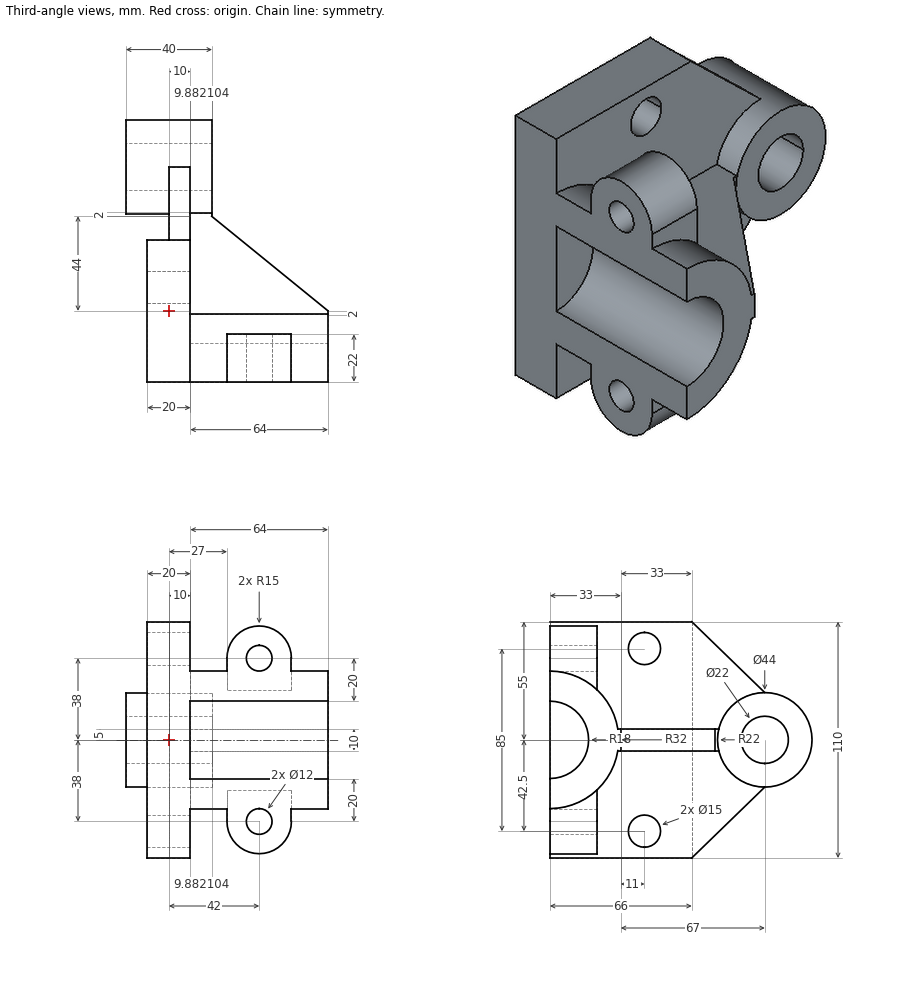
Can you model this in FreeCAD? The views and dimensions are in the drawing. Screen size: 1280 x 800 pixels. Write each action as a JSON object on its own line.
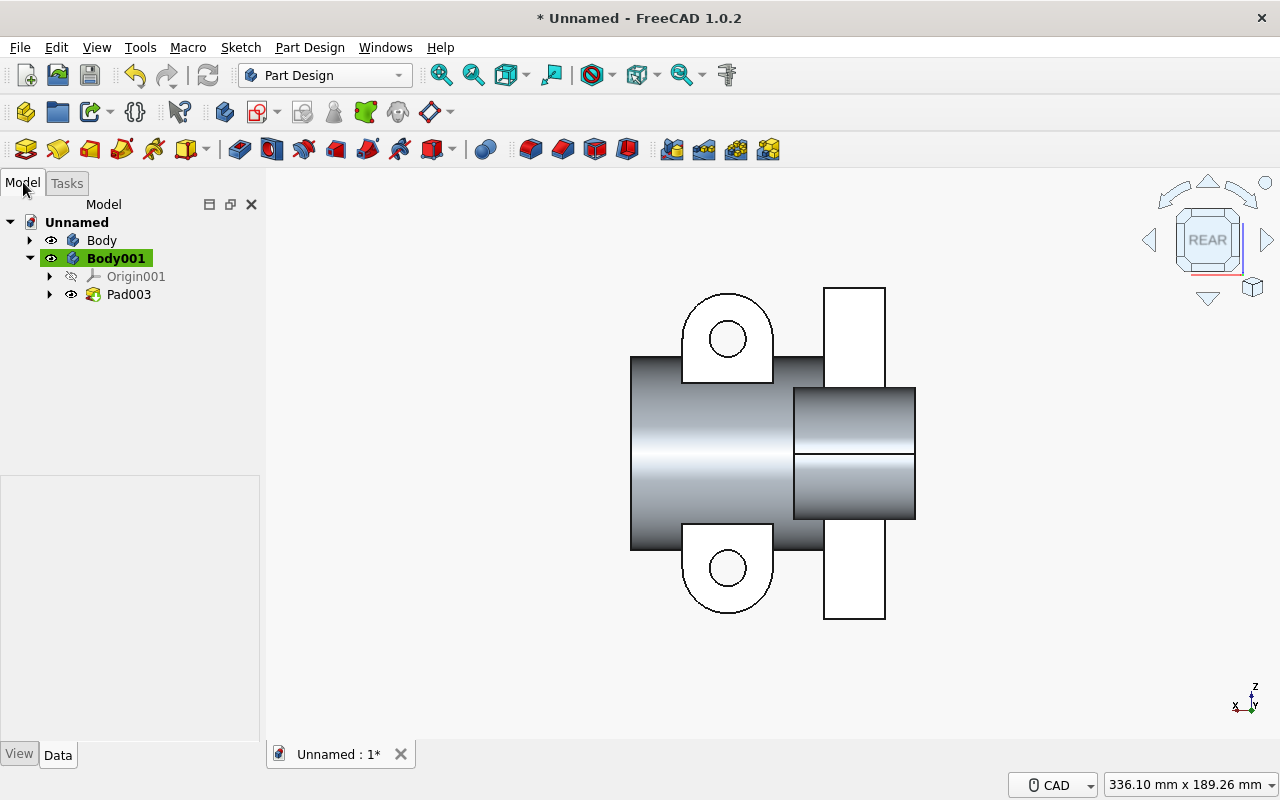
{"action": "double_click", "coordinate": [96, 240]}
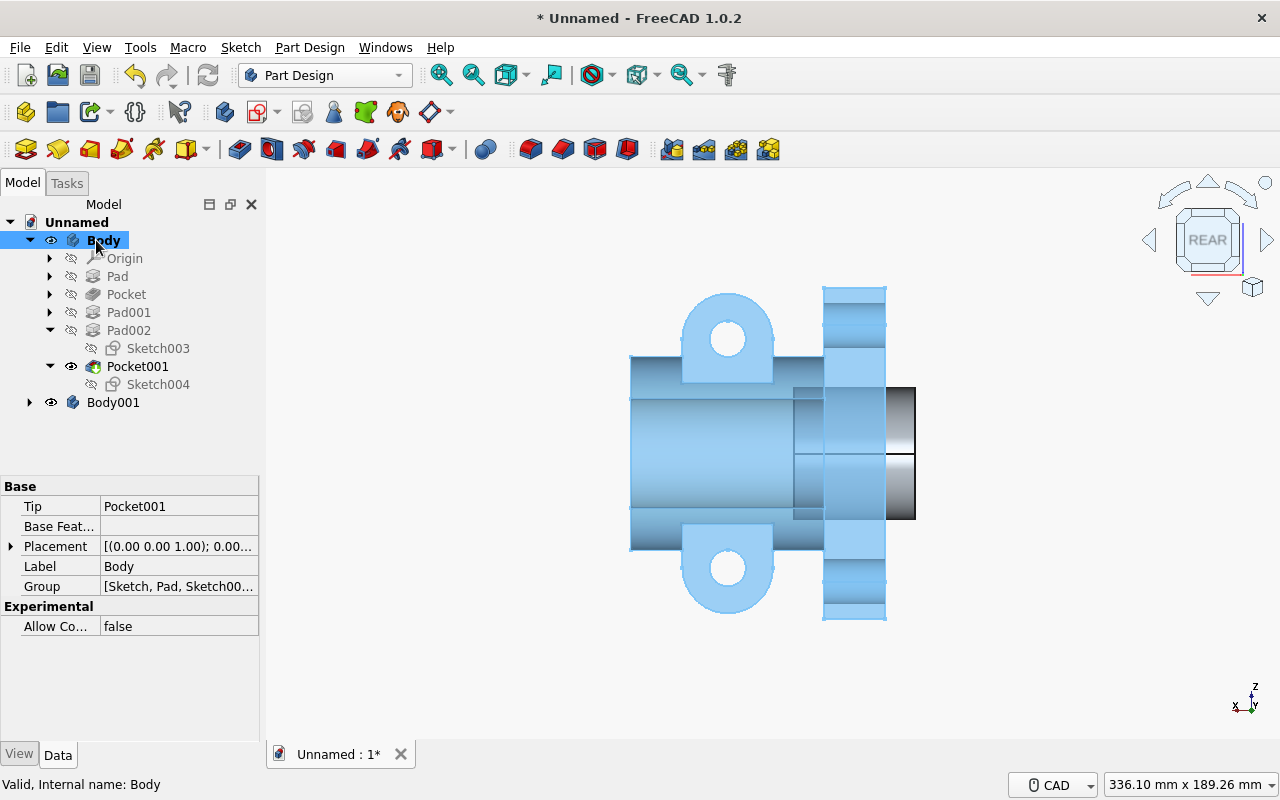
{"action": "left_click", "coordinate": [96, 240]}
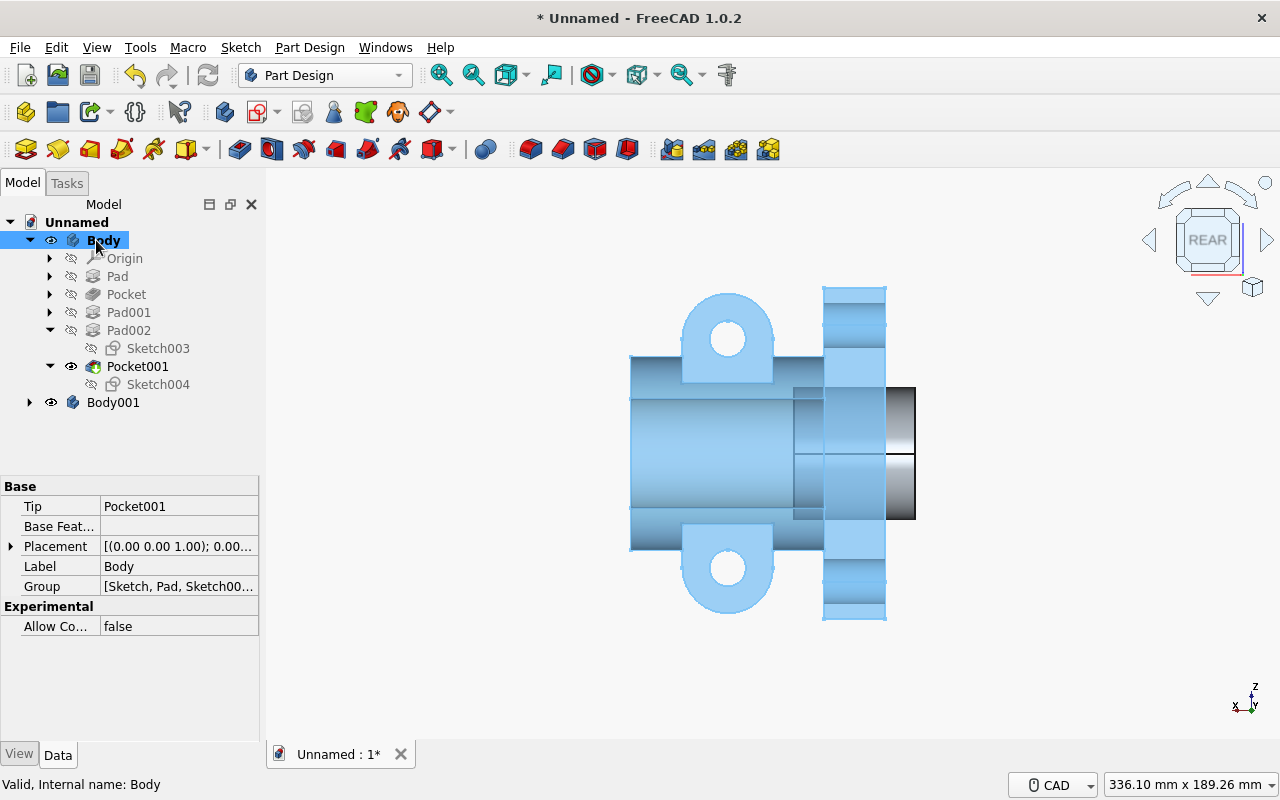
{"action": "left_click", "coordinate": [146, 626]}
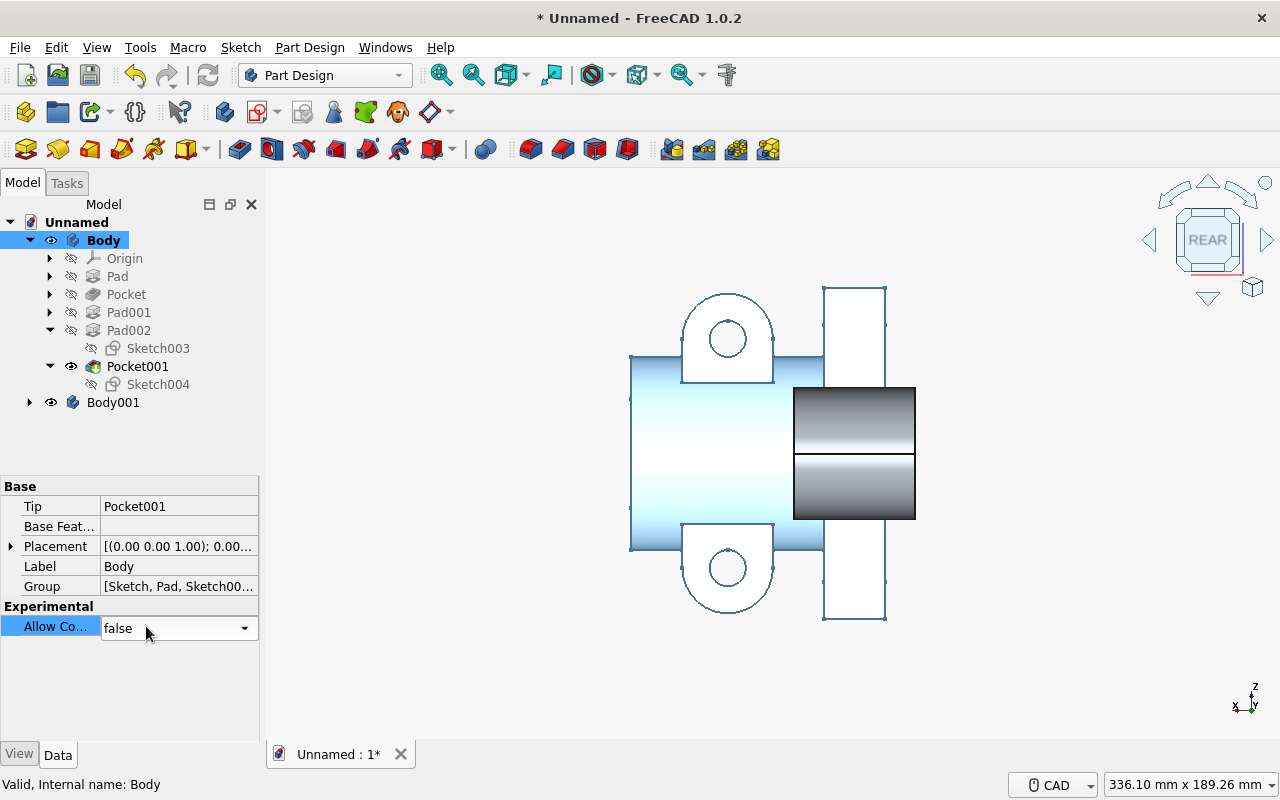
{"action": "left_click", "coordinate": [146, 626]}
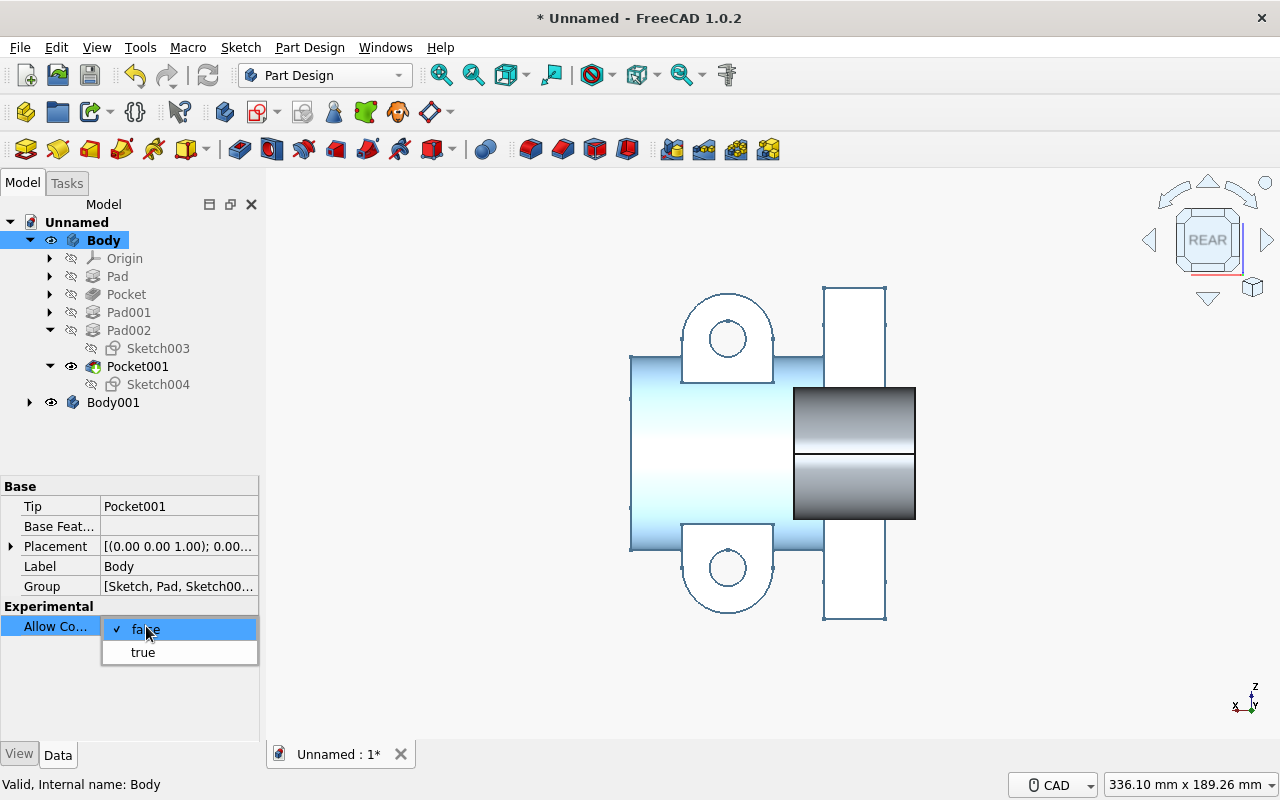
{"action": "left_click", "coordinate": [179, 652]}
{"action": "key", "text": "Return"}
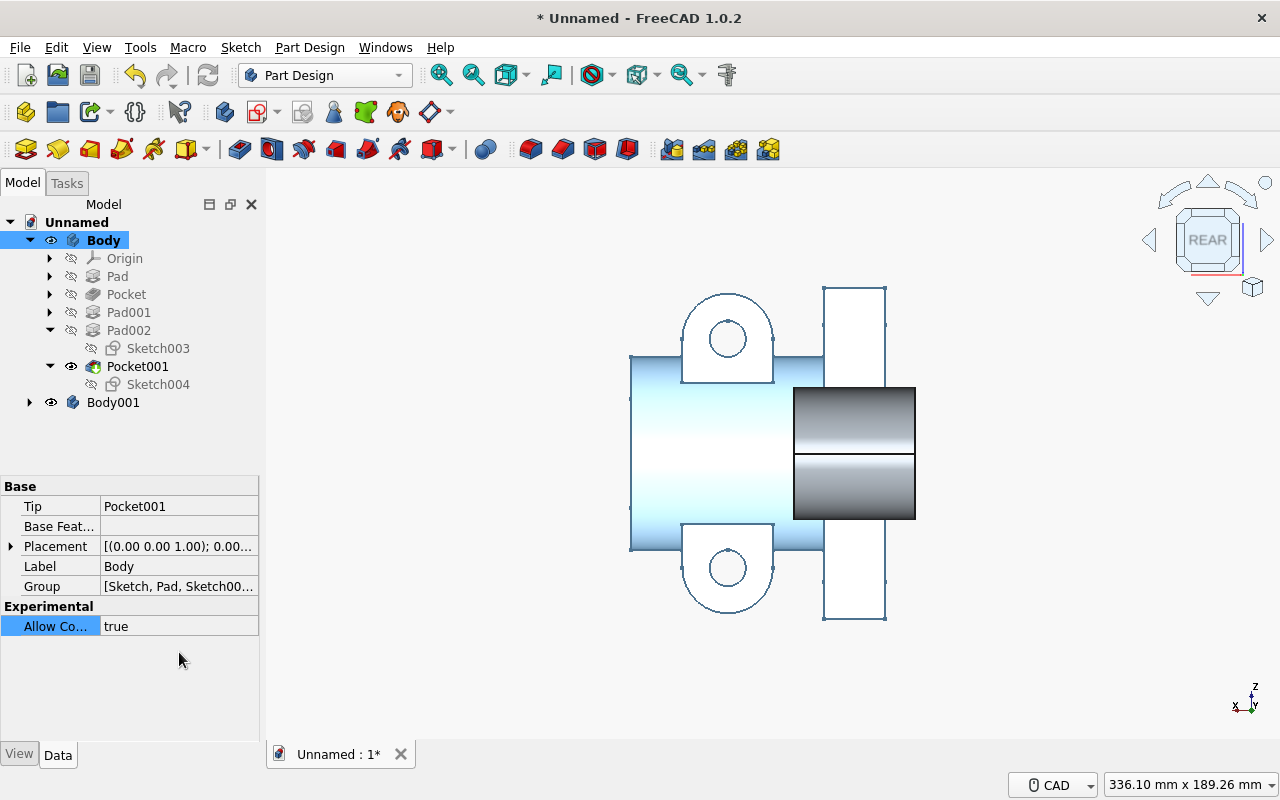
{"action": "left_click", "coordinate": [96, 402]}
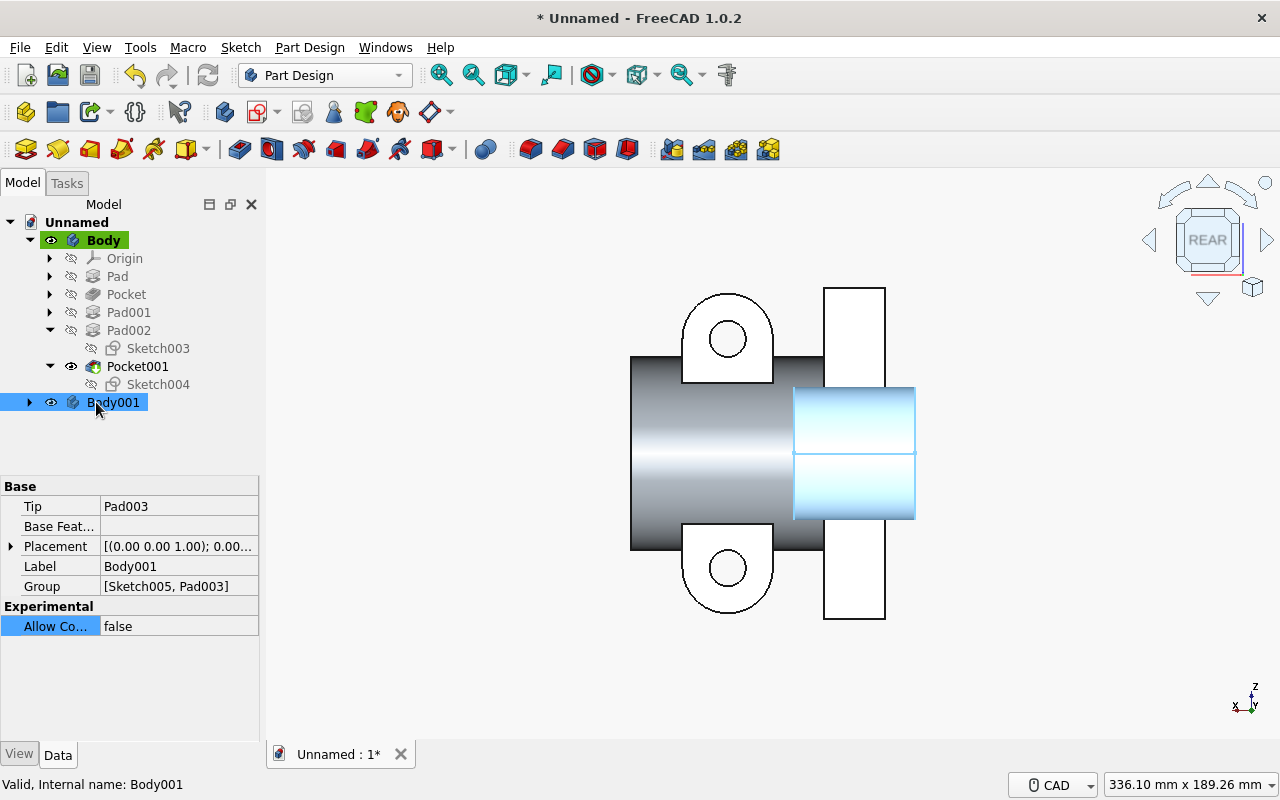
{"action": "left_click", "coordinate": [486, 150]}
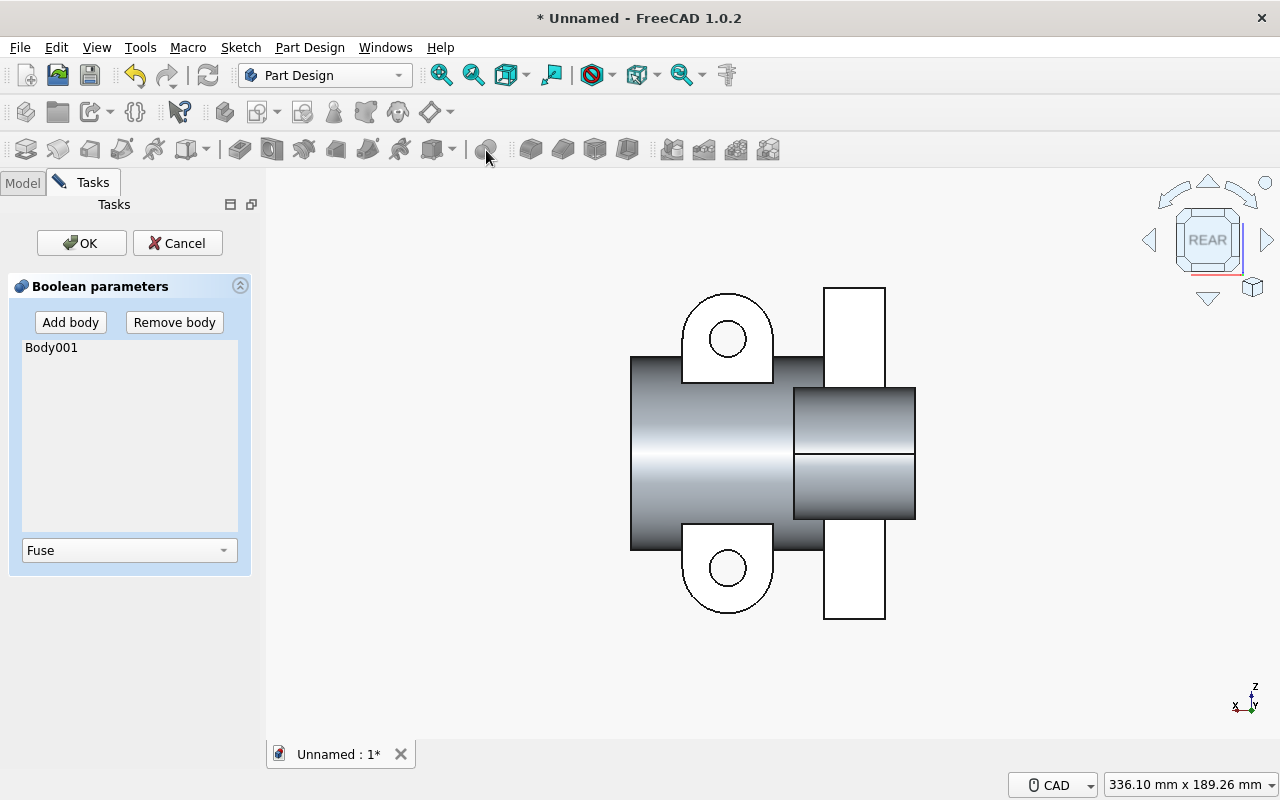
{"action": "left_click", "coordinate": [82, 243]}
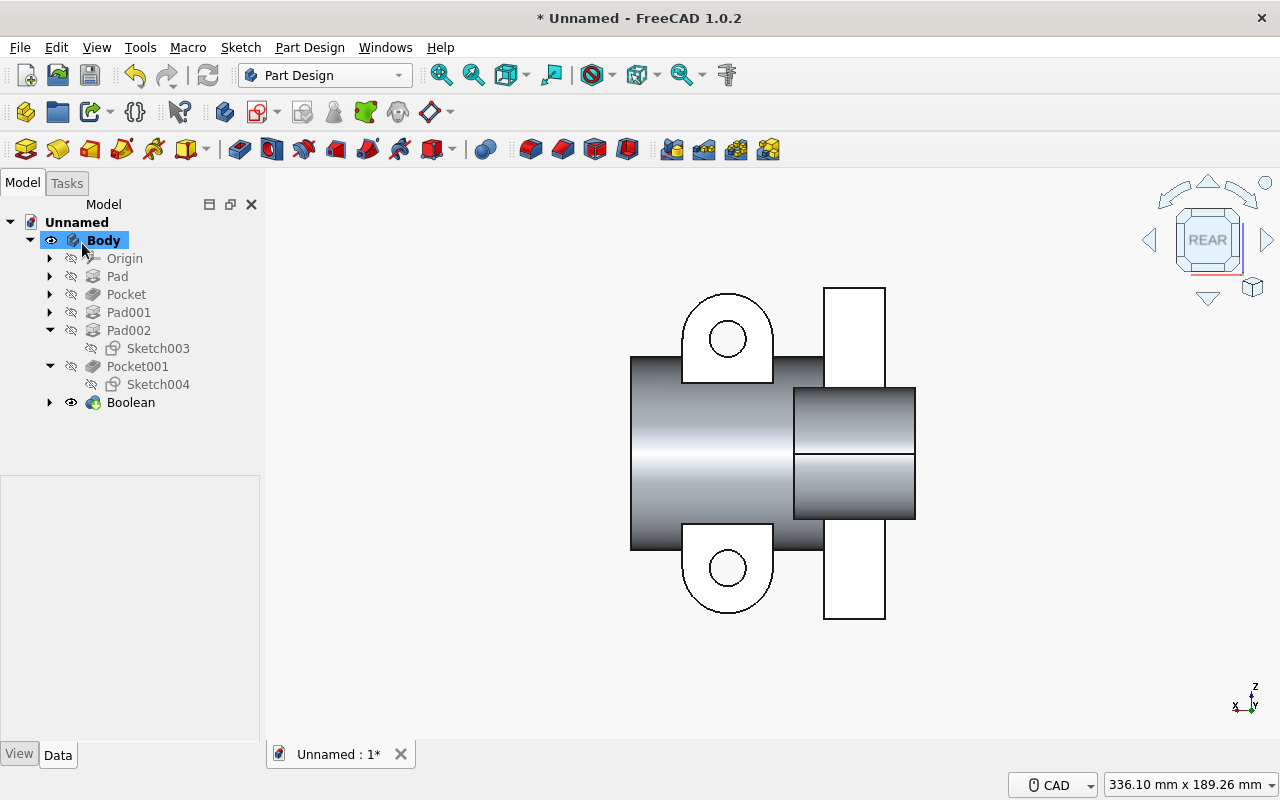
{"action": "key", "text": "0"}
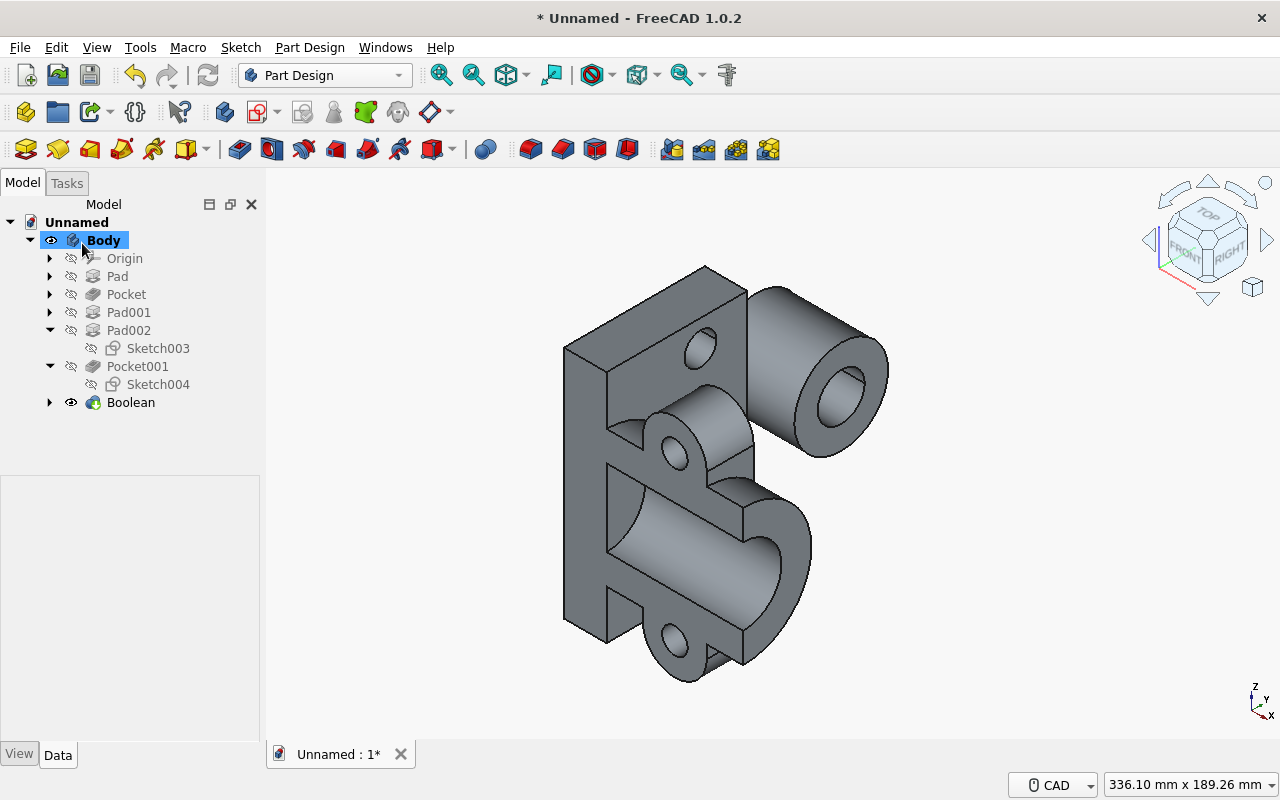
{"action": "left_click", "coordinate": [677, 389]}